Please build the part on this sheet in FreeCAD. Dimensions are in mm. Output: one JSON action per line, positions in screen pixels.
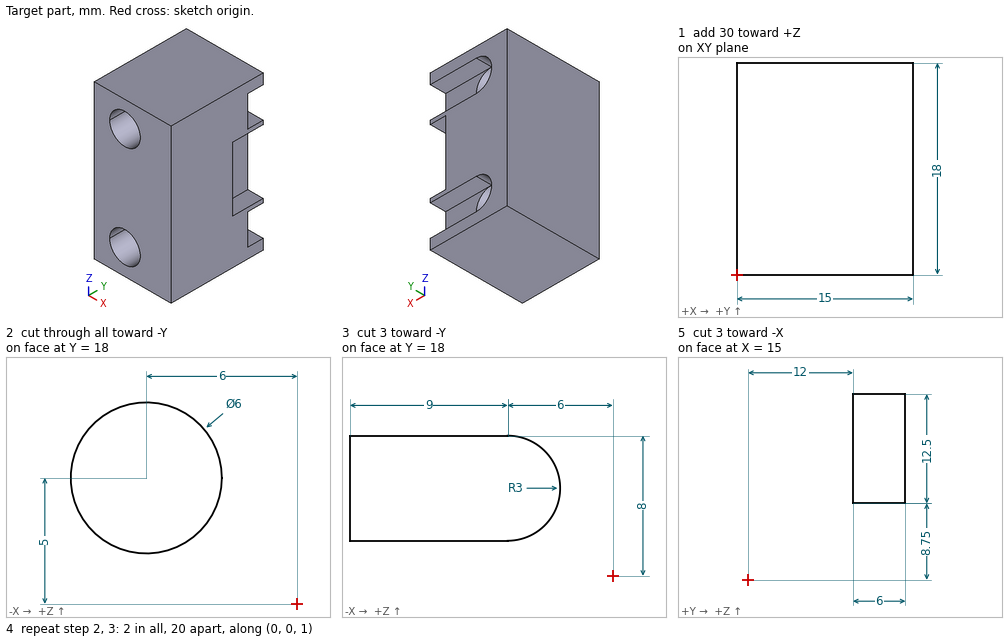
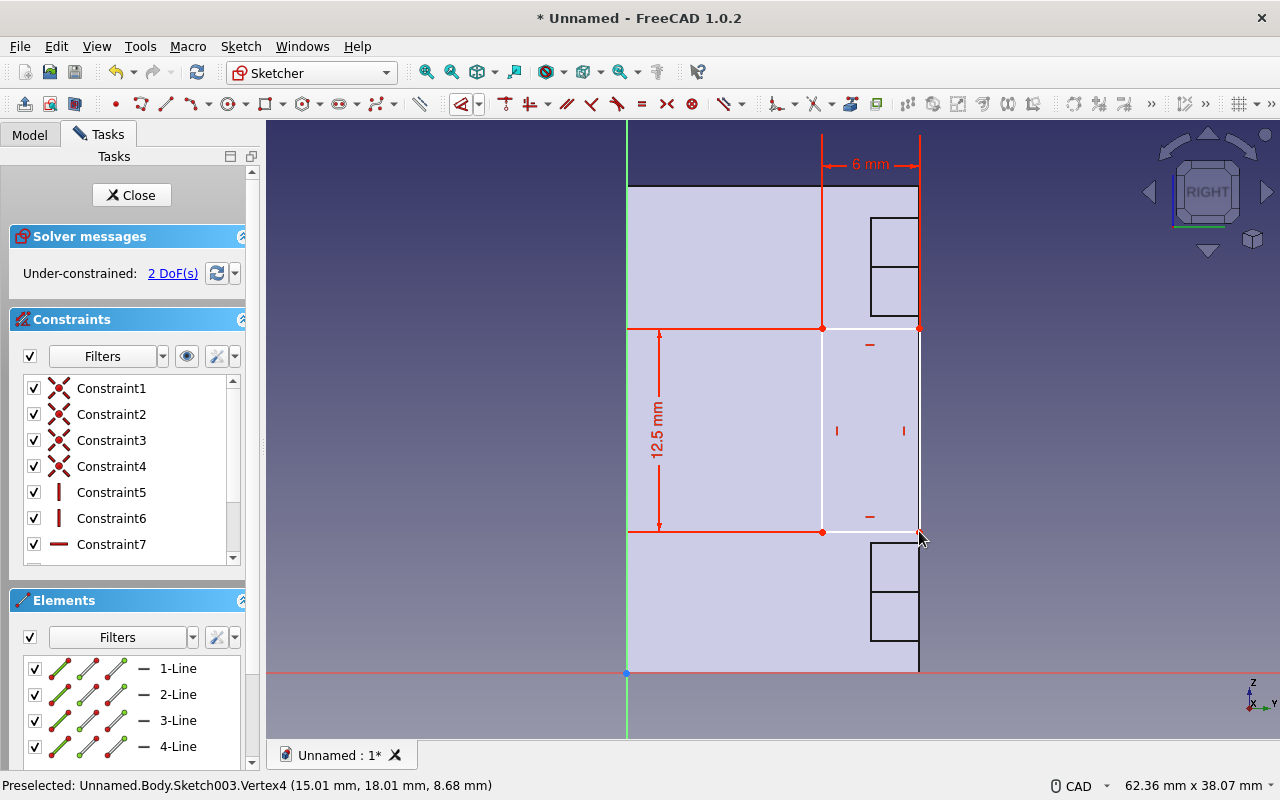
{"action": "left_click", "coordinate": [822, 329]}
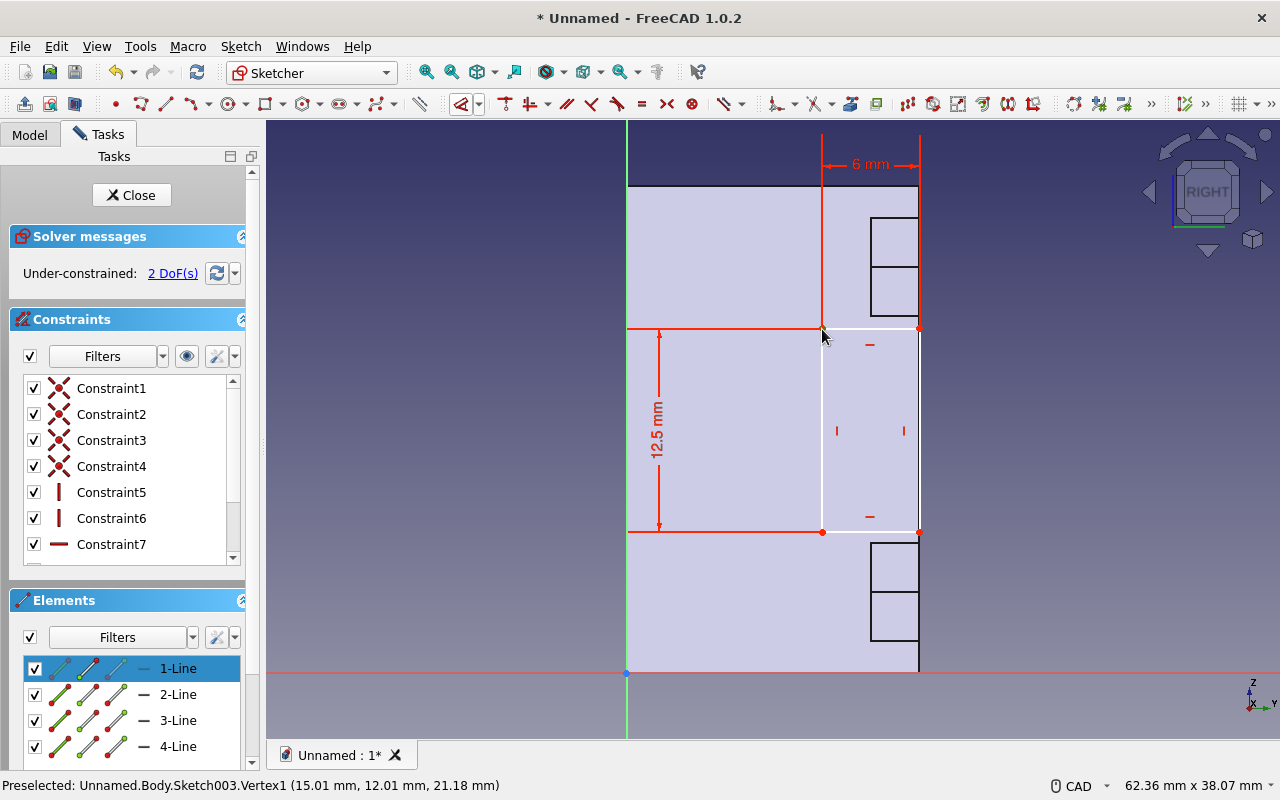
{"action": "left_click", "coordinate": [478, 104]}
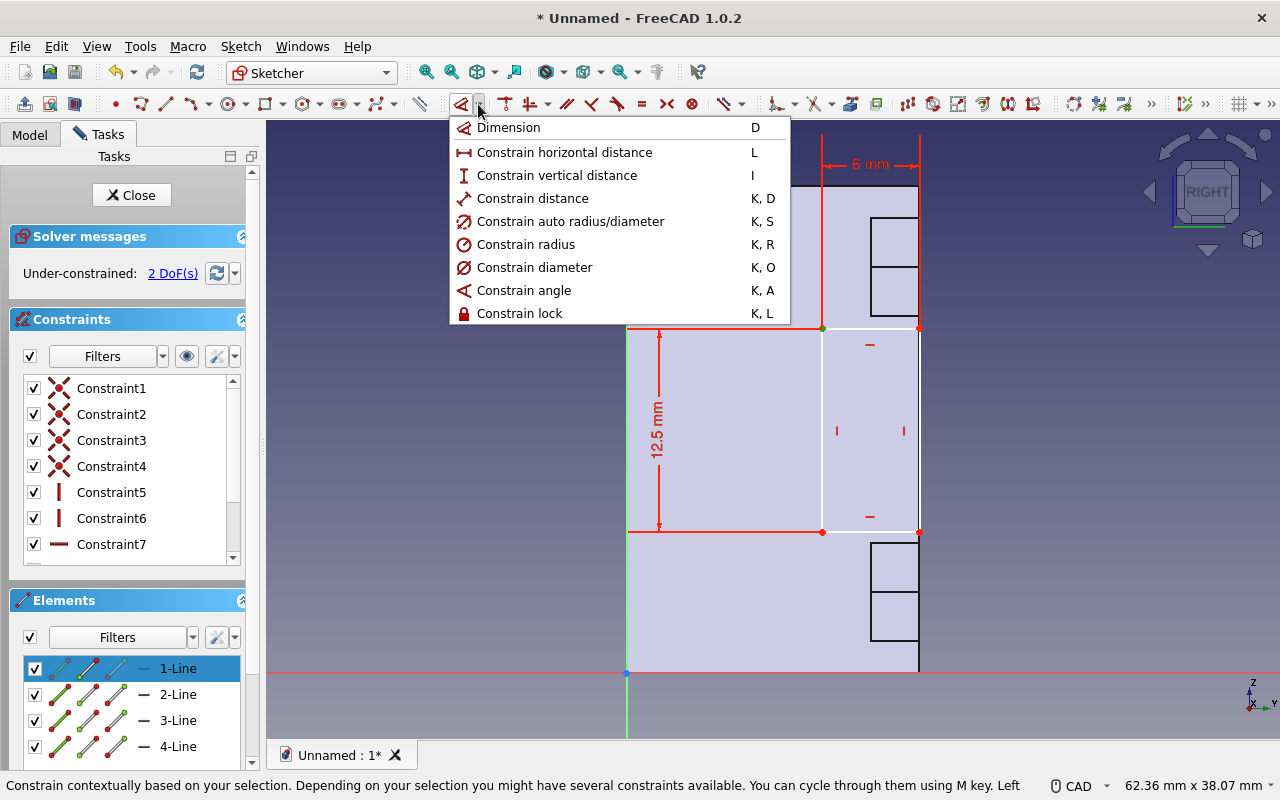
{"action": "left_click", "coordinate": [620, 152]}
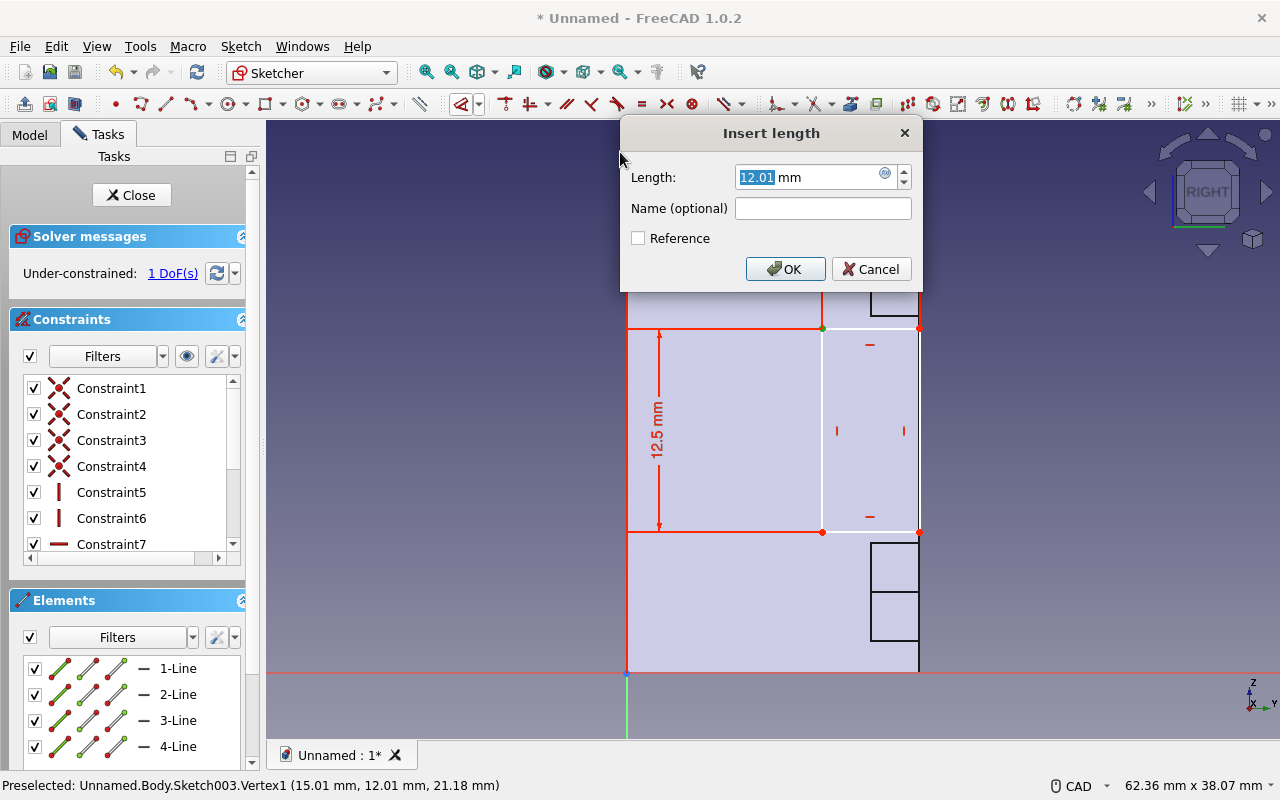
{"action": "type", "text": "12"}
{"action": "key", "text": "Return"}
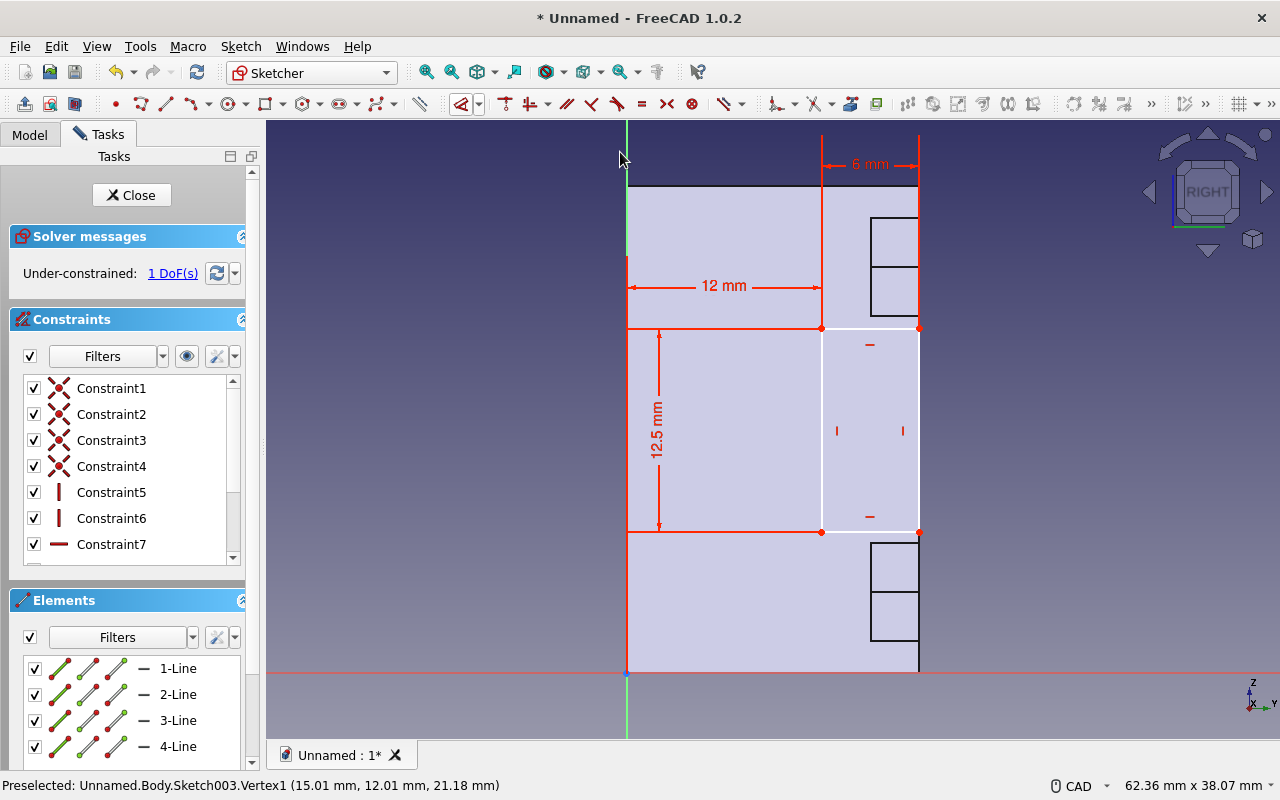
{"action": "left_click", "coordinate": [822, 532]}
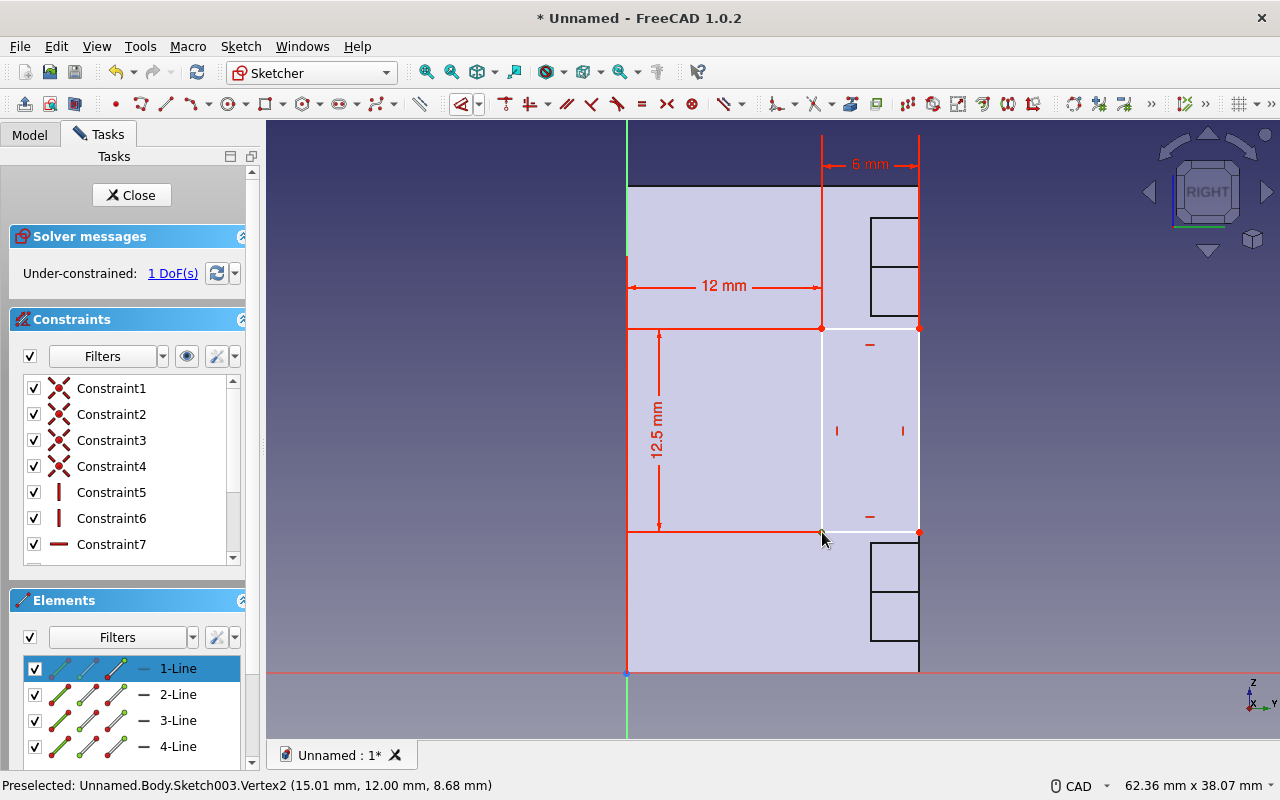
{"action": "key", "text": "i"}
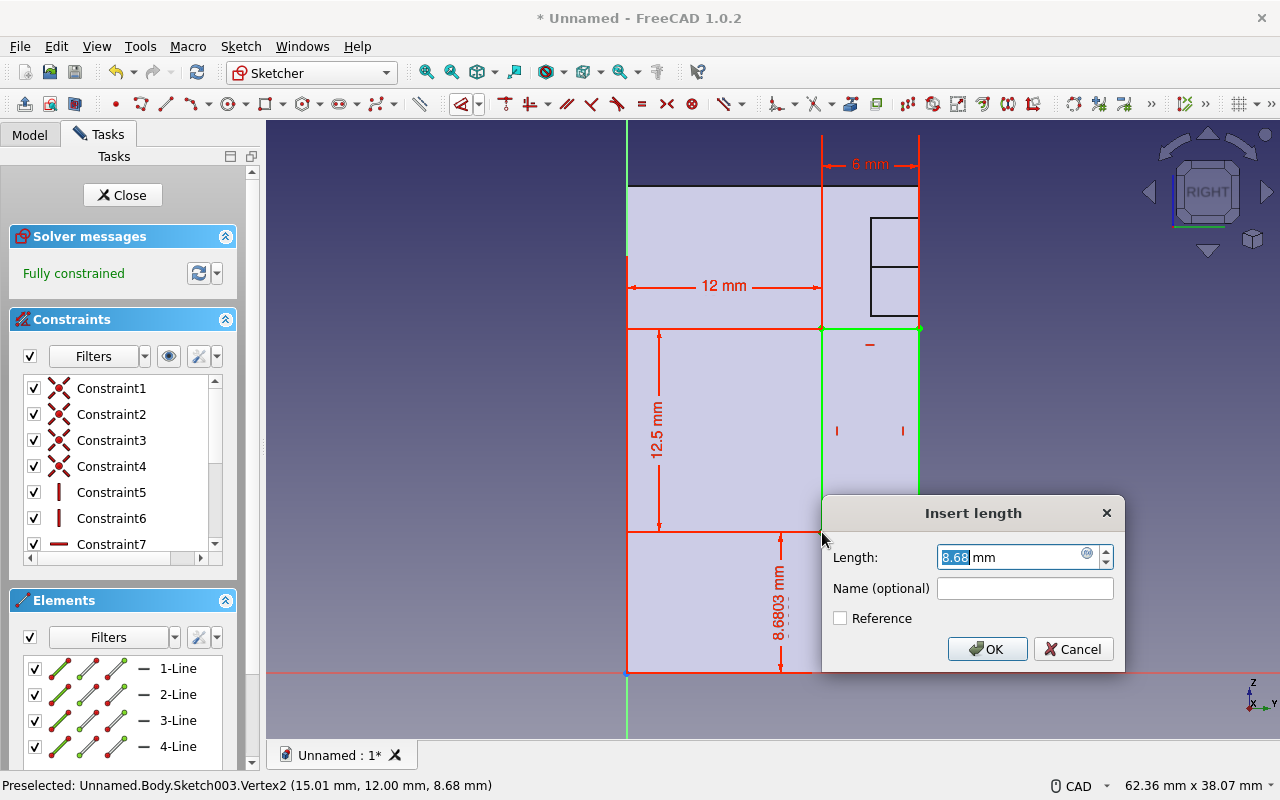
{"action": "type", "text": "8.75"}
{"action": "key", "text": "Return"}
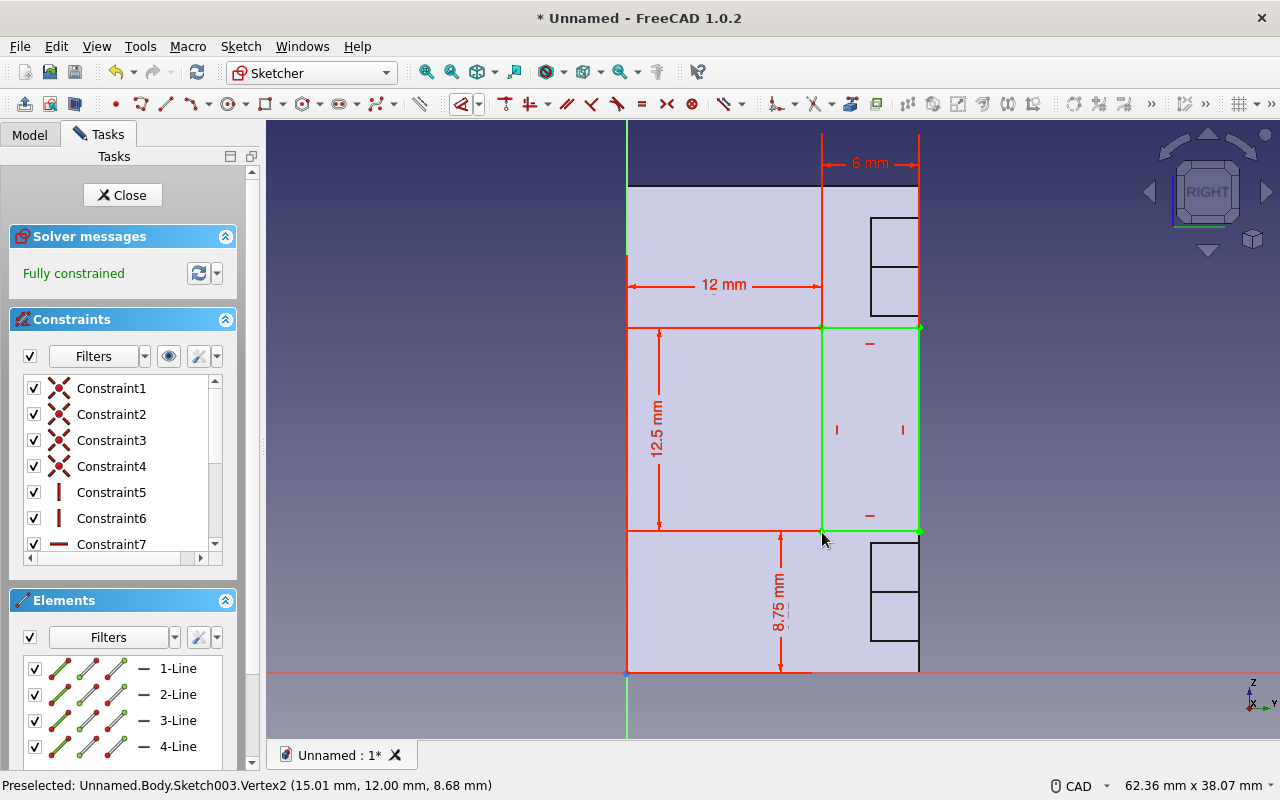
{"action": "left_click", "coordinate": [123, 195]}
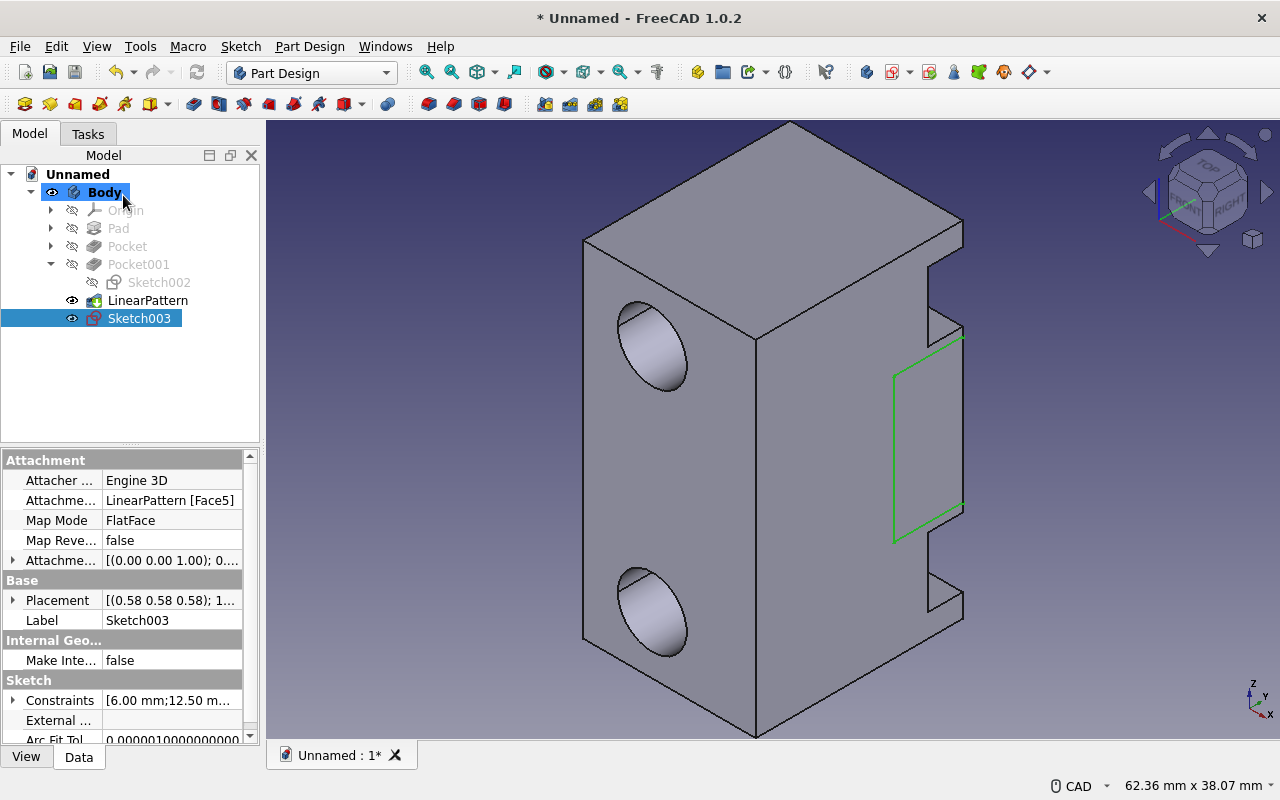
{"action": "left_click", "coordinate": [194, 104]}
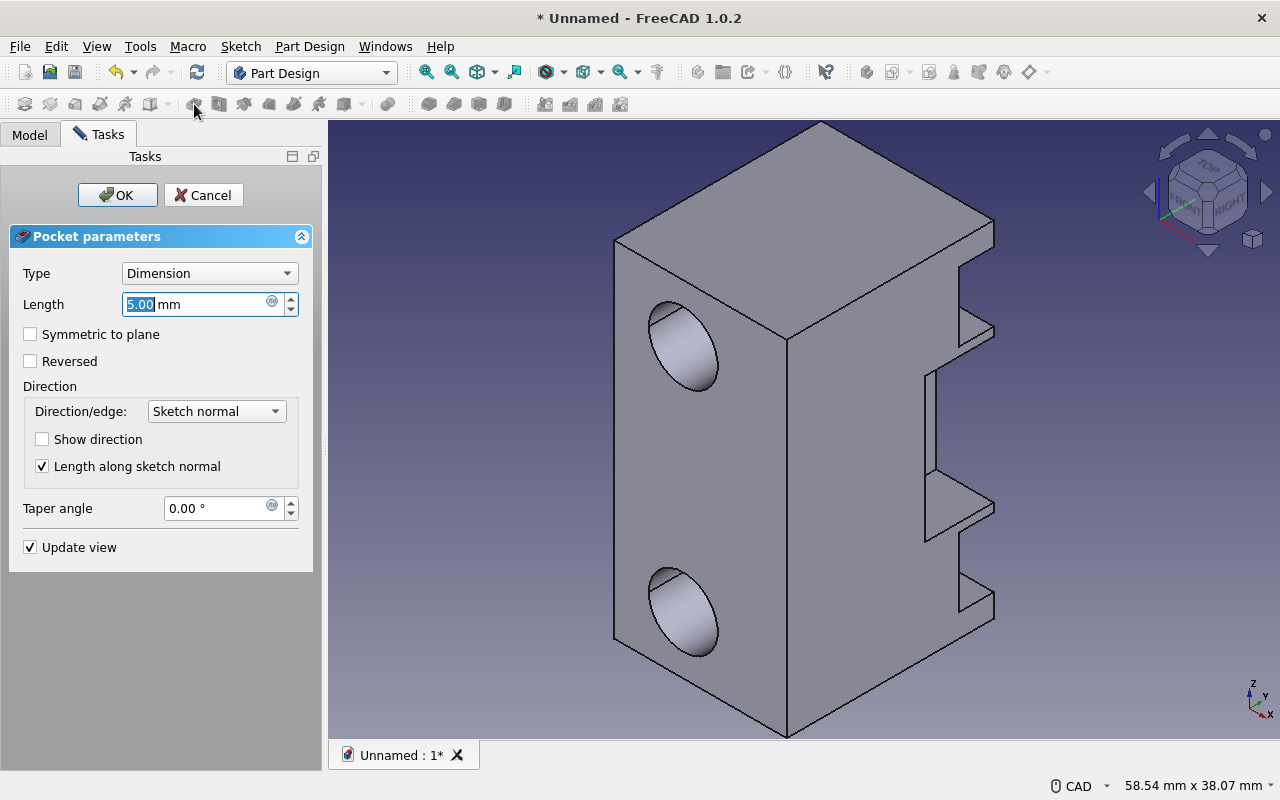
{"action": "type", "text": "3"}
{"action": "key", "text": "Tab"}